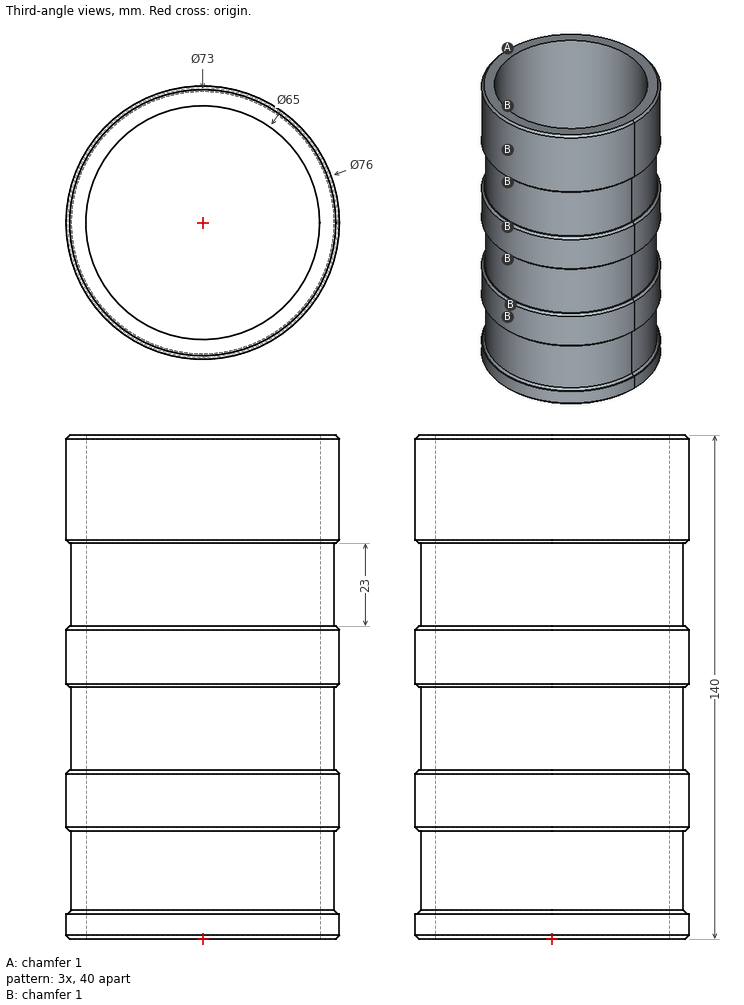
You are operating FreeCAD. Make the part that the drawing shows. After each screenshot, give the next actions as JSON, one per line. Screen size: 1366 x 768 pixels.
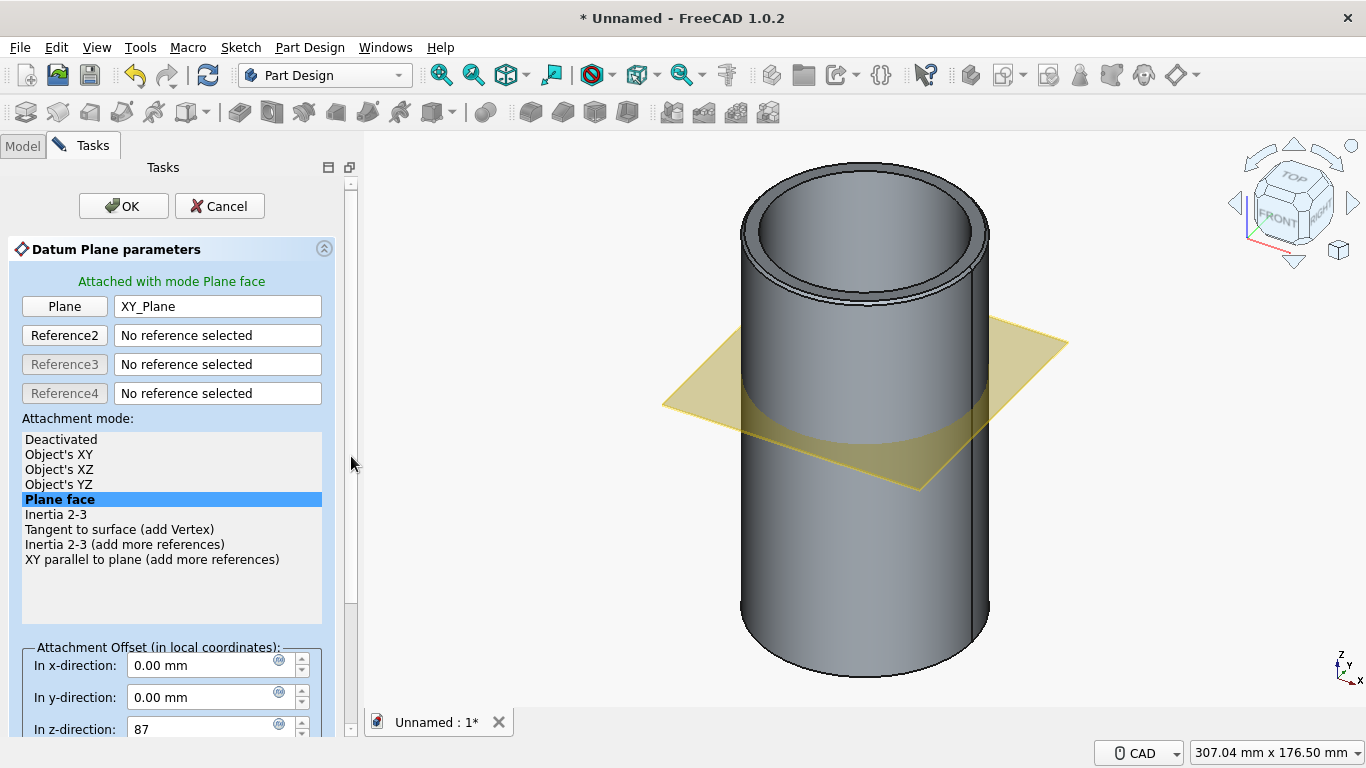
{"action": "left_click", "coordinate": [124, 206]}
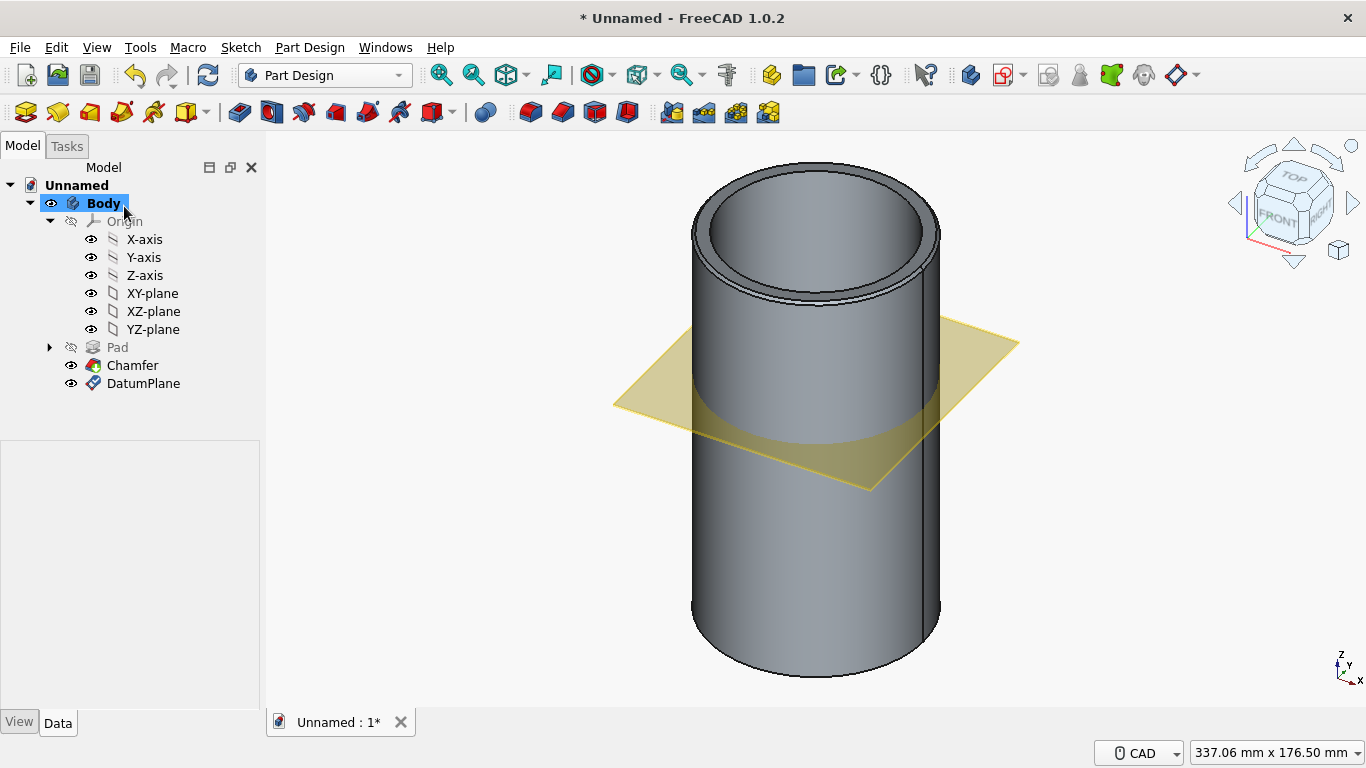
{"action": "left_click", "coordinate": [116, 383]}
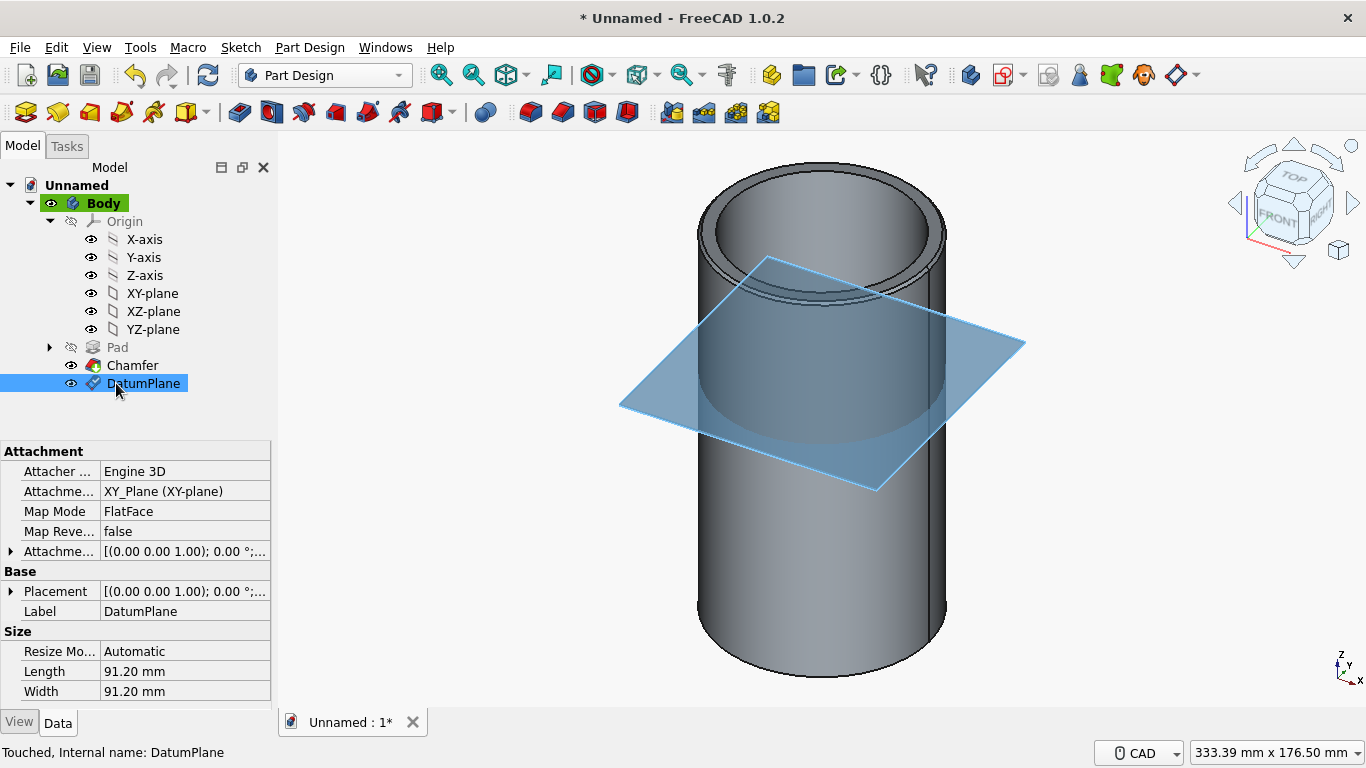
{"action": "left_click", "coordinate": [1004, 76]}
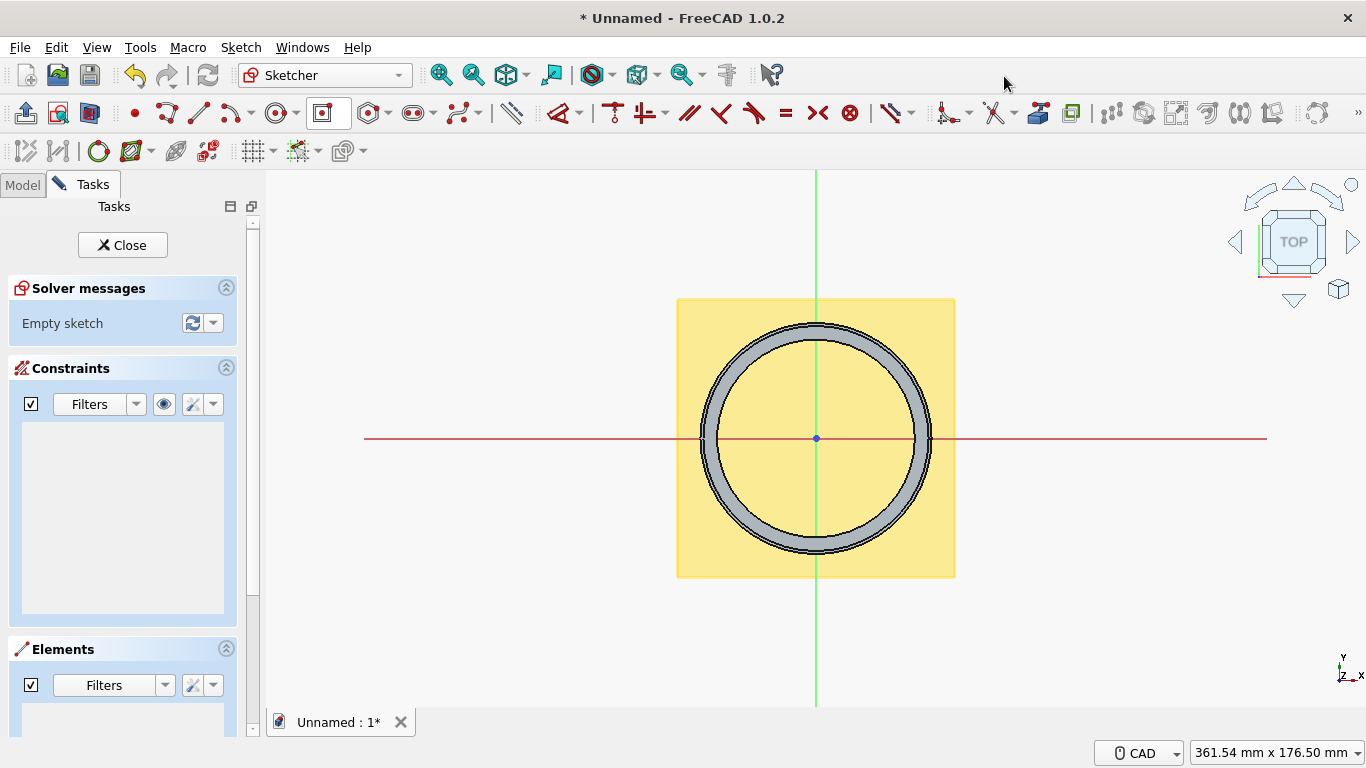
{"action": "key", "text": "q s"}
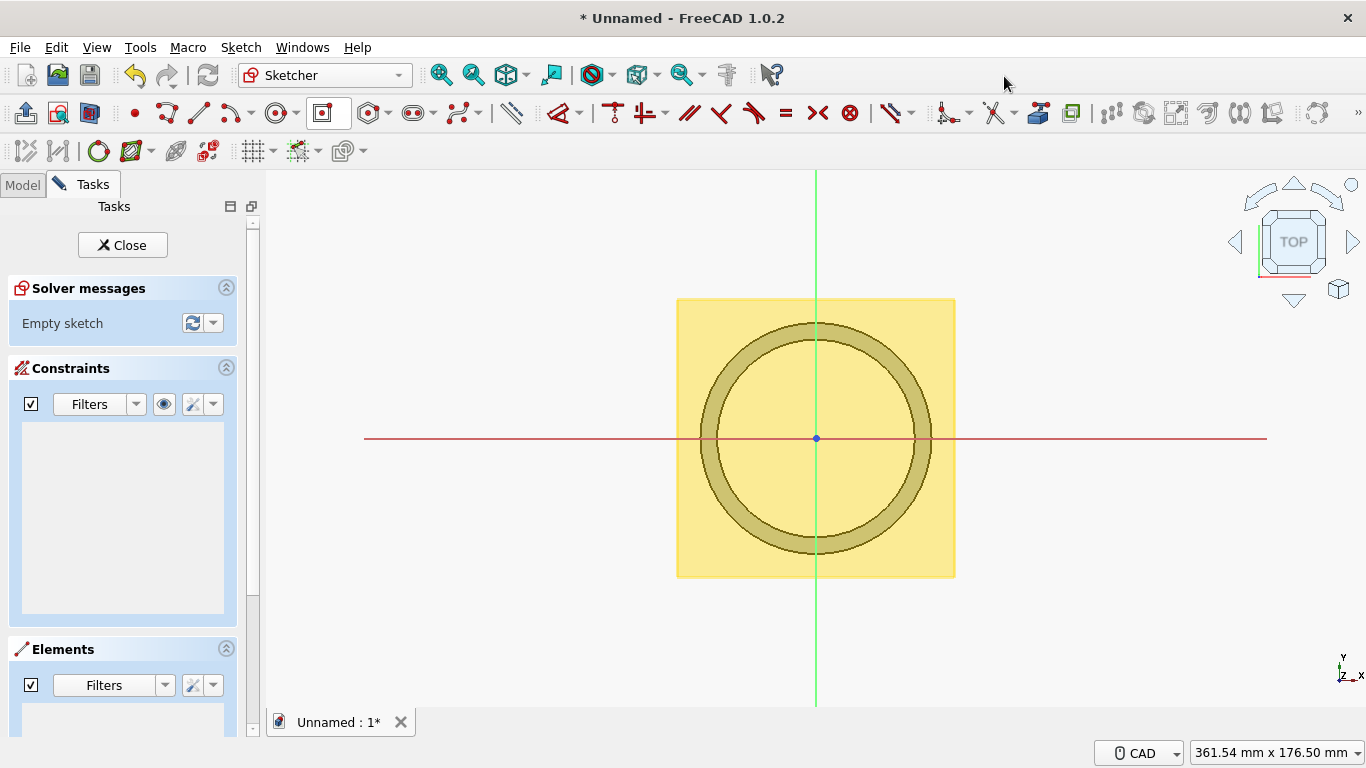
{"action": "scroll", "coordinate": [955, 439], "scroll_direction": "up", "scroll_amount": 2}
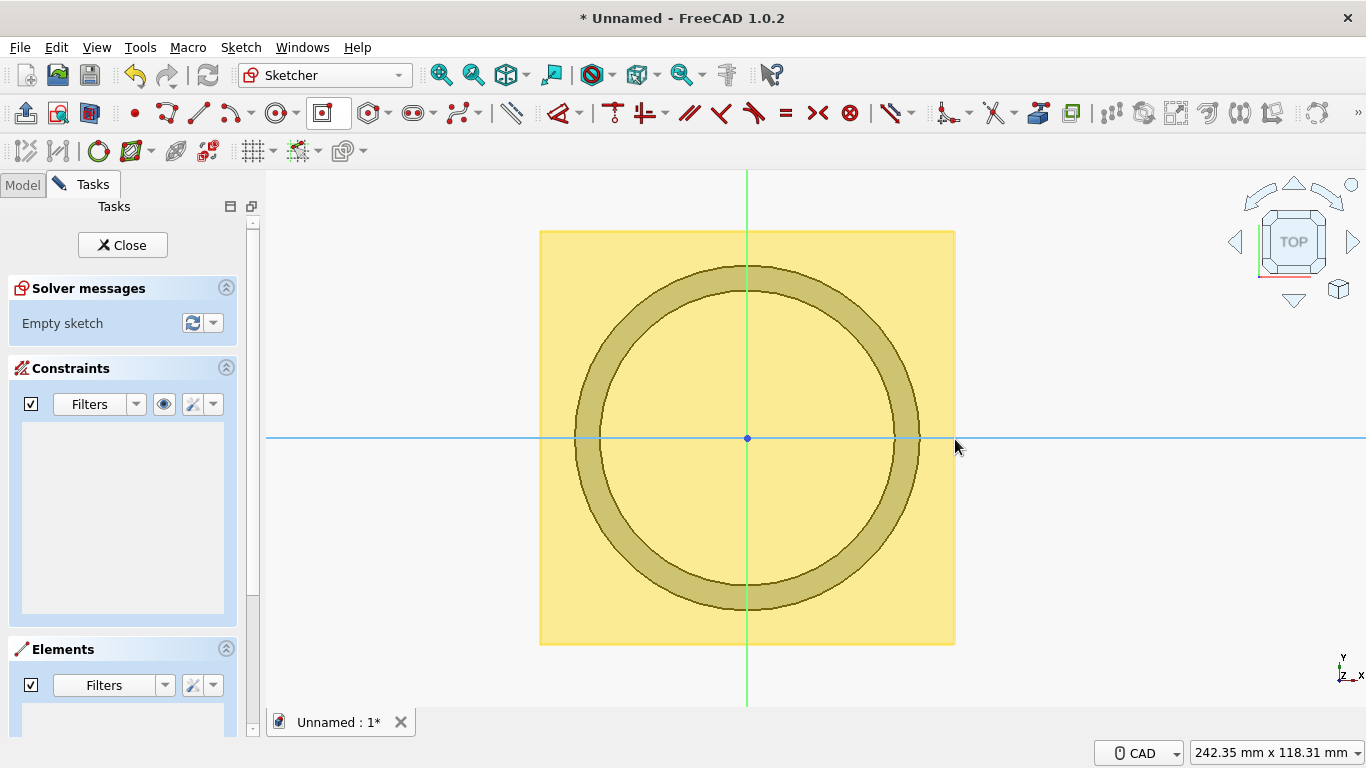
{"action": "key", "text": "g c"}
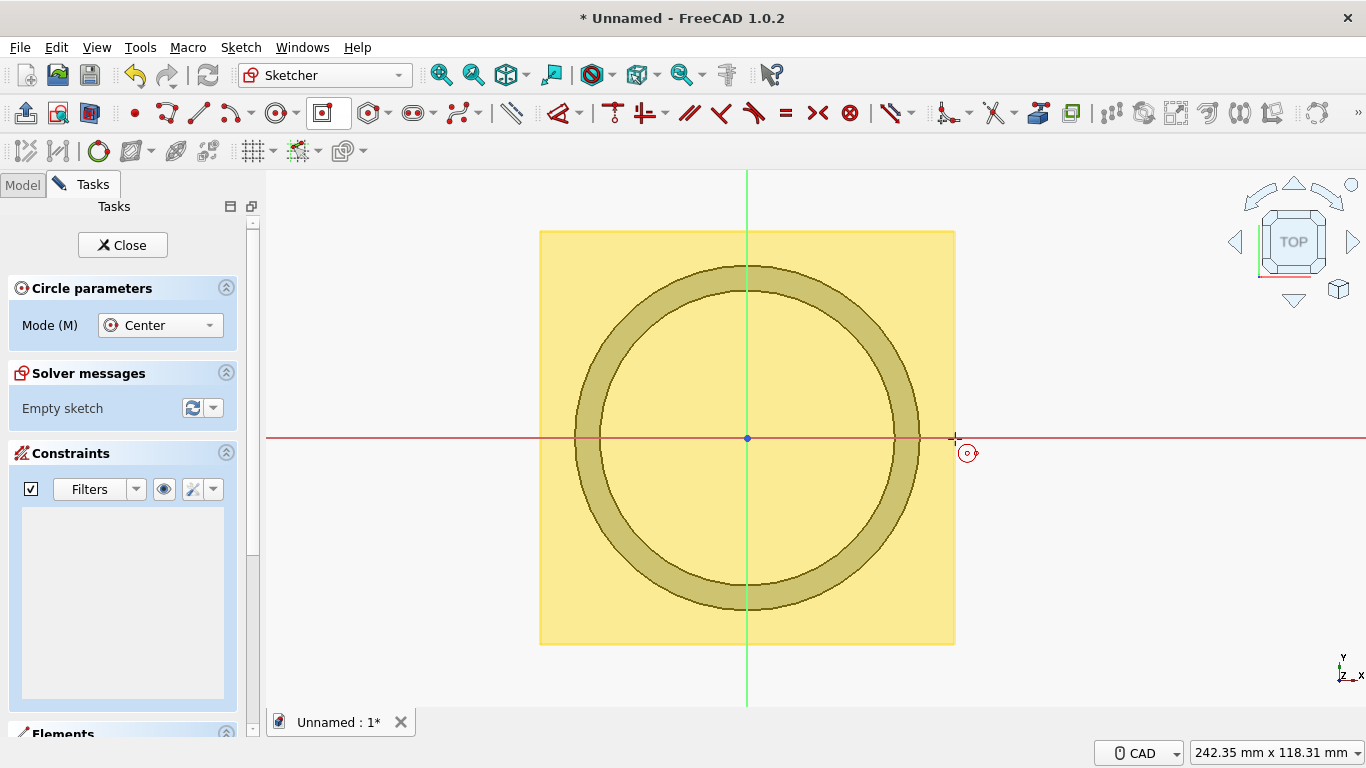
{"action": "left_click", "coordinate": [747, 438]}
{"action": "left_click", "coordinate": [869, 316]}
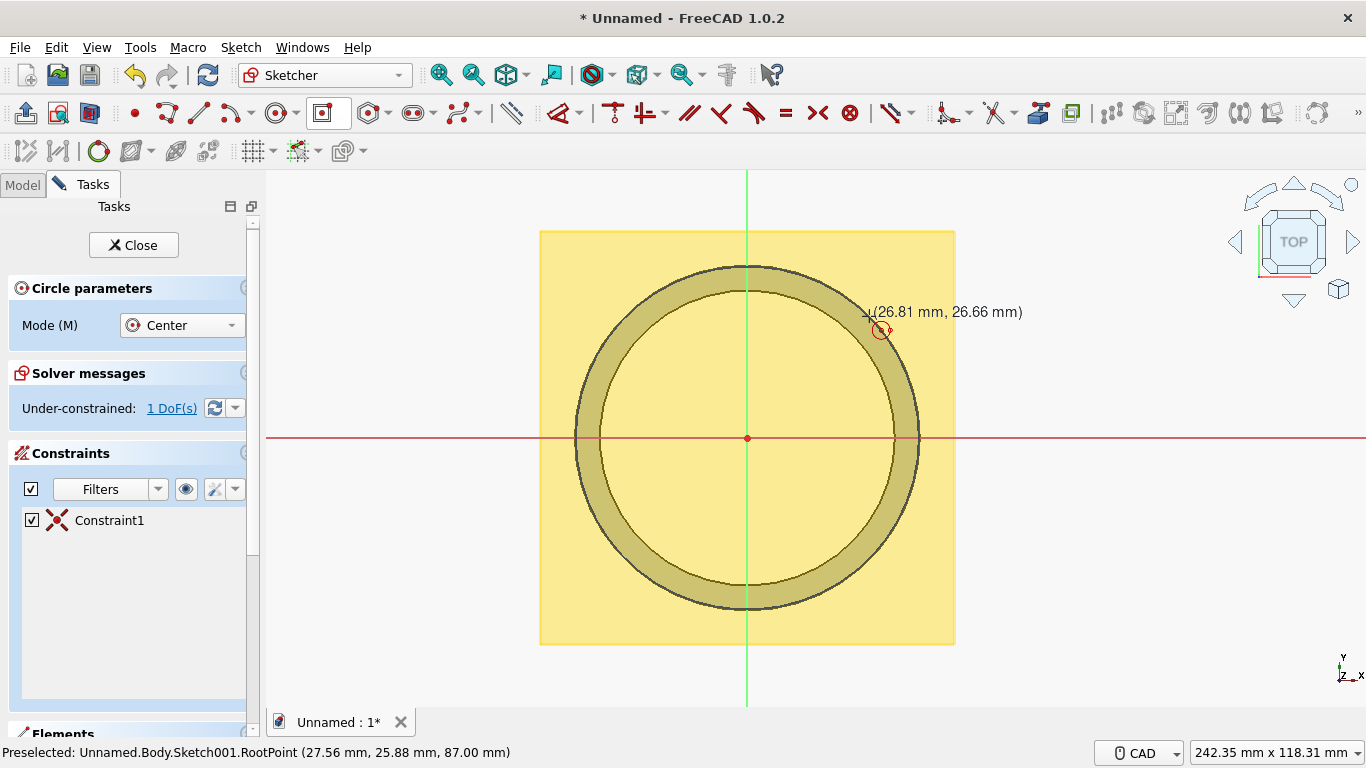
{"action": "left_click", "coordinate": [747, 438]}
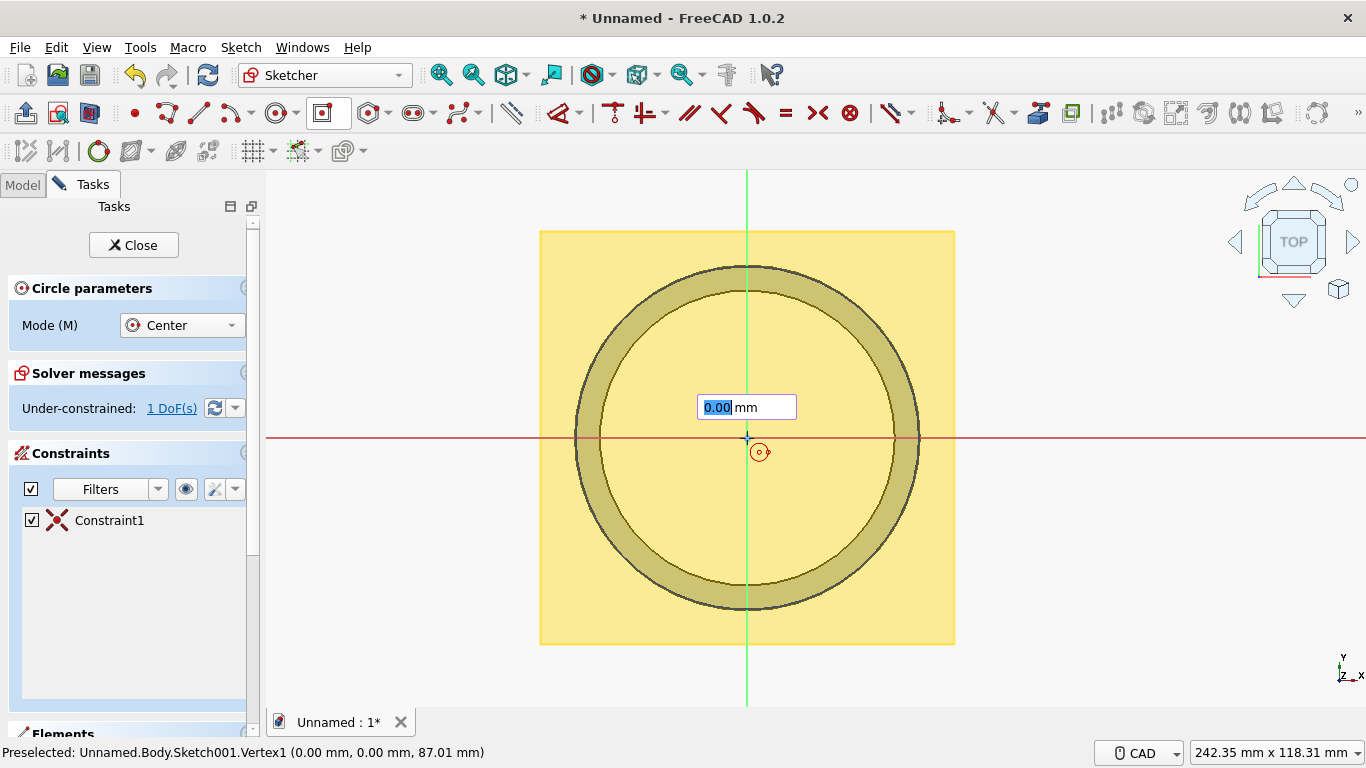
{"action": "scroll", "coordinate": [804, 282], "scroll_direction": "up", "scroll_amount": 5}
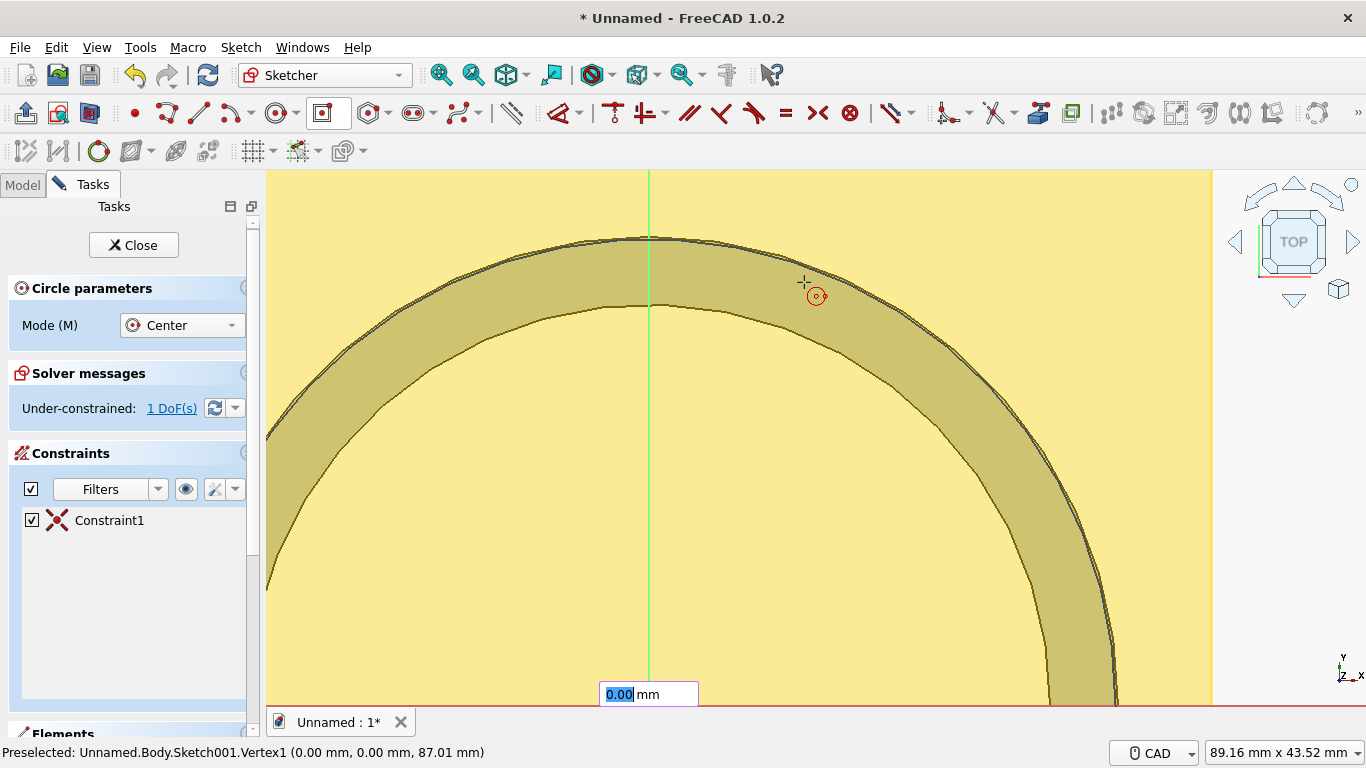
{"action": "left_click", "coordinate": [803, 283]}
{"action": "key", "text": "Escape"}